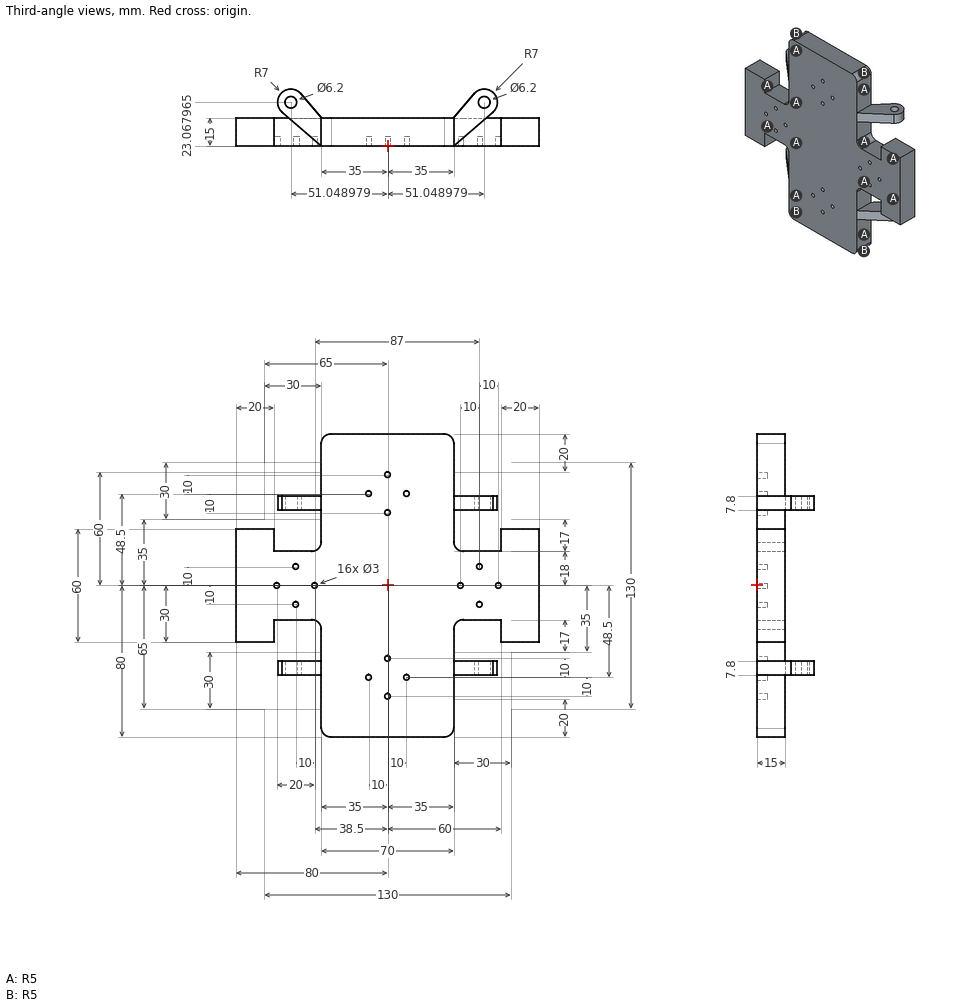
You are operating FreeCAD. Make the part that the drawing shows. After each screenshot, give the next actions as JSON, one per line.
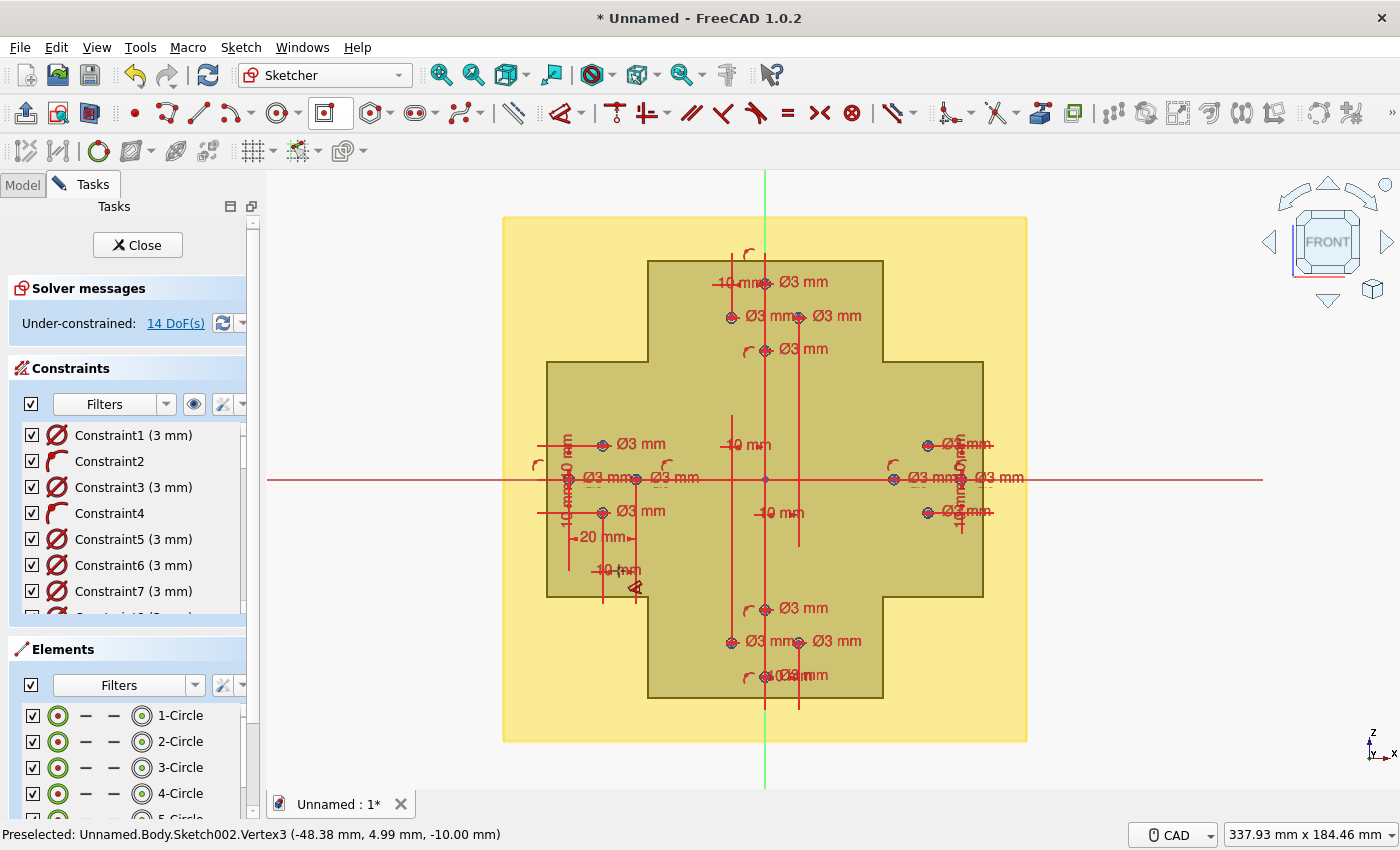
{"action": "left_click", "coordinate": [636, 480]}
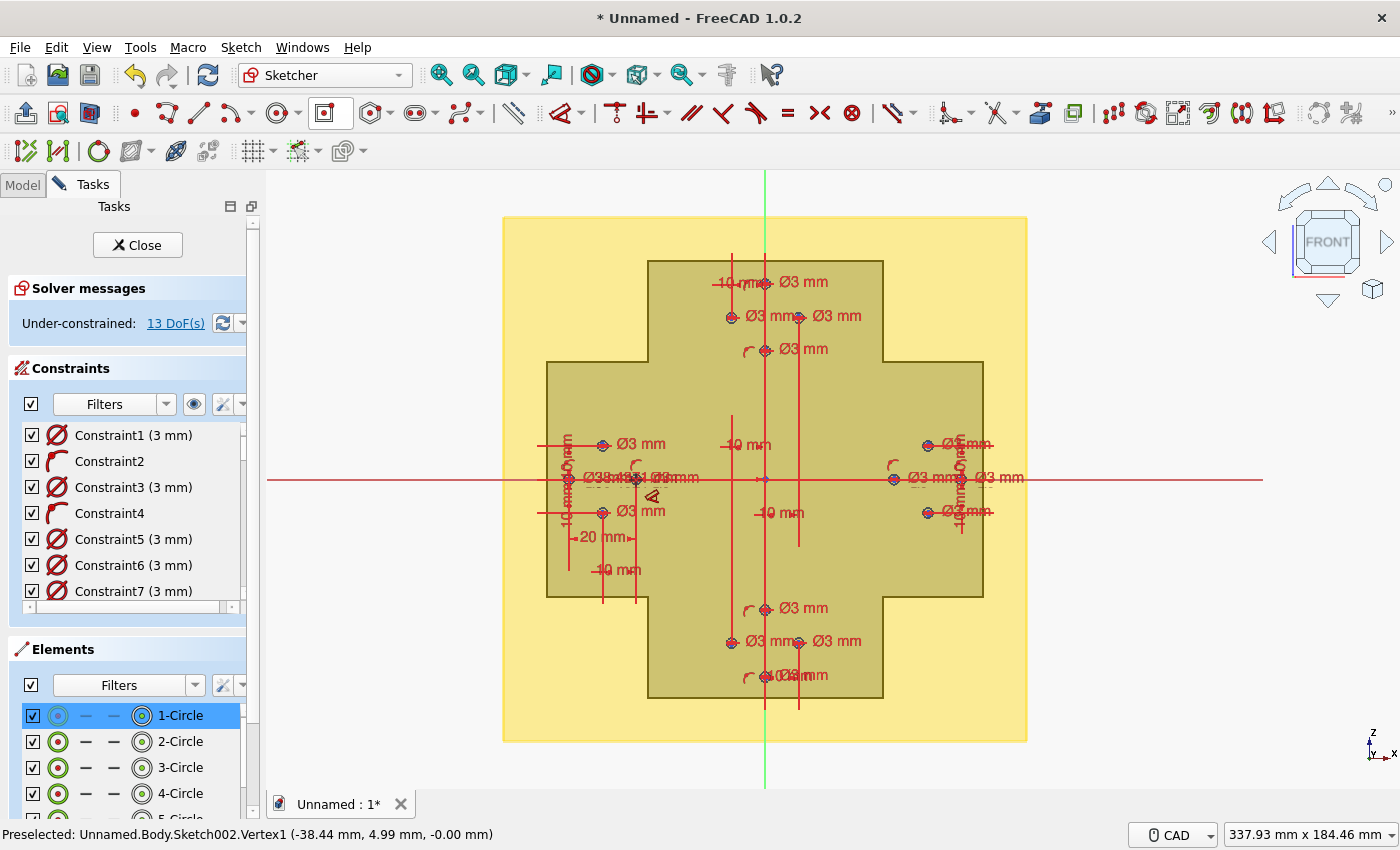
{"action": "left_click", "coordinate": [603, 446]}
{"action": "left_click", "coordinate": [619, 412]}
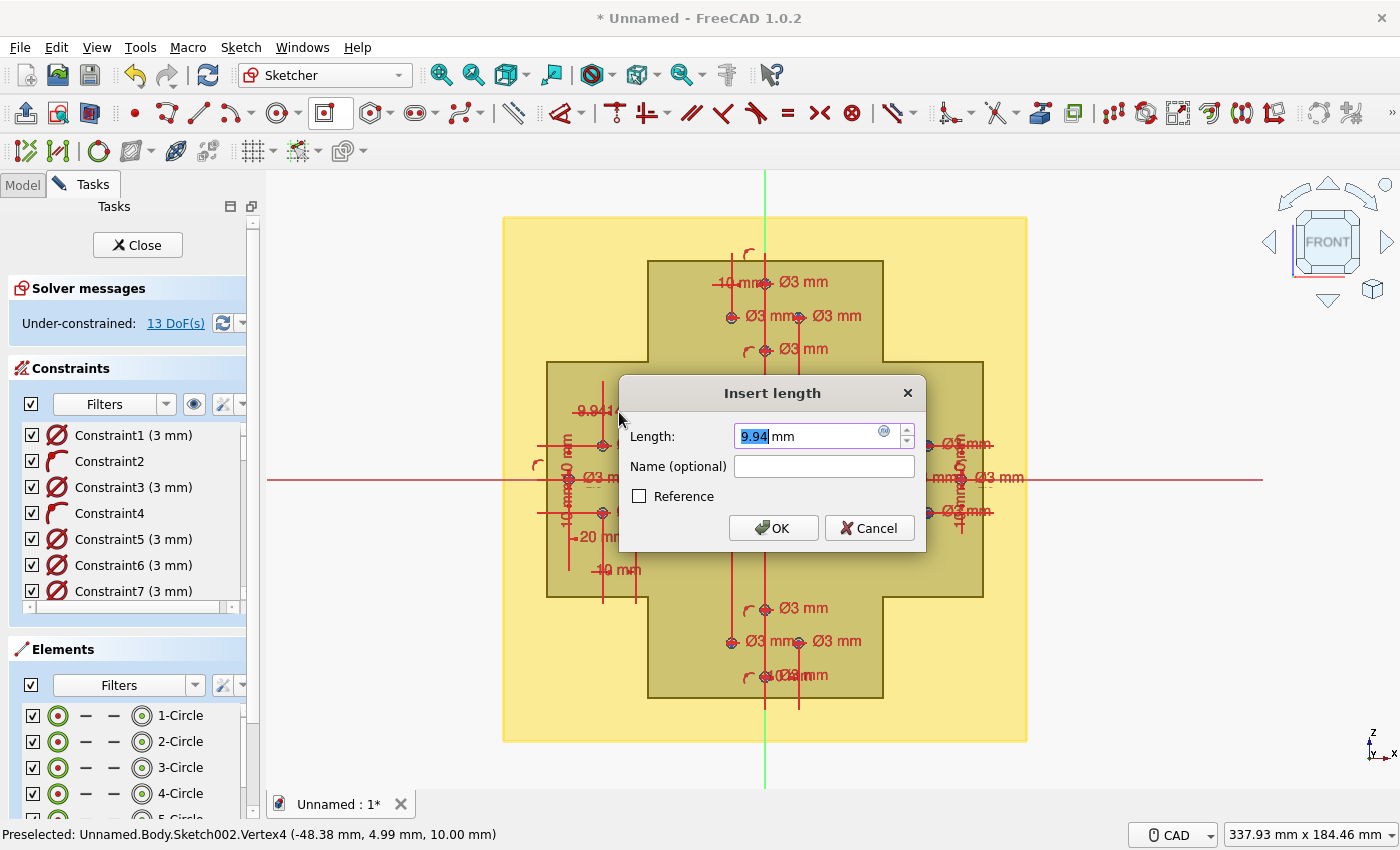
{"action": "type", "text": "10"}
{"action": "key", "text": "Return"}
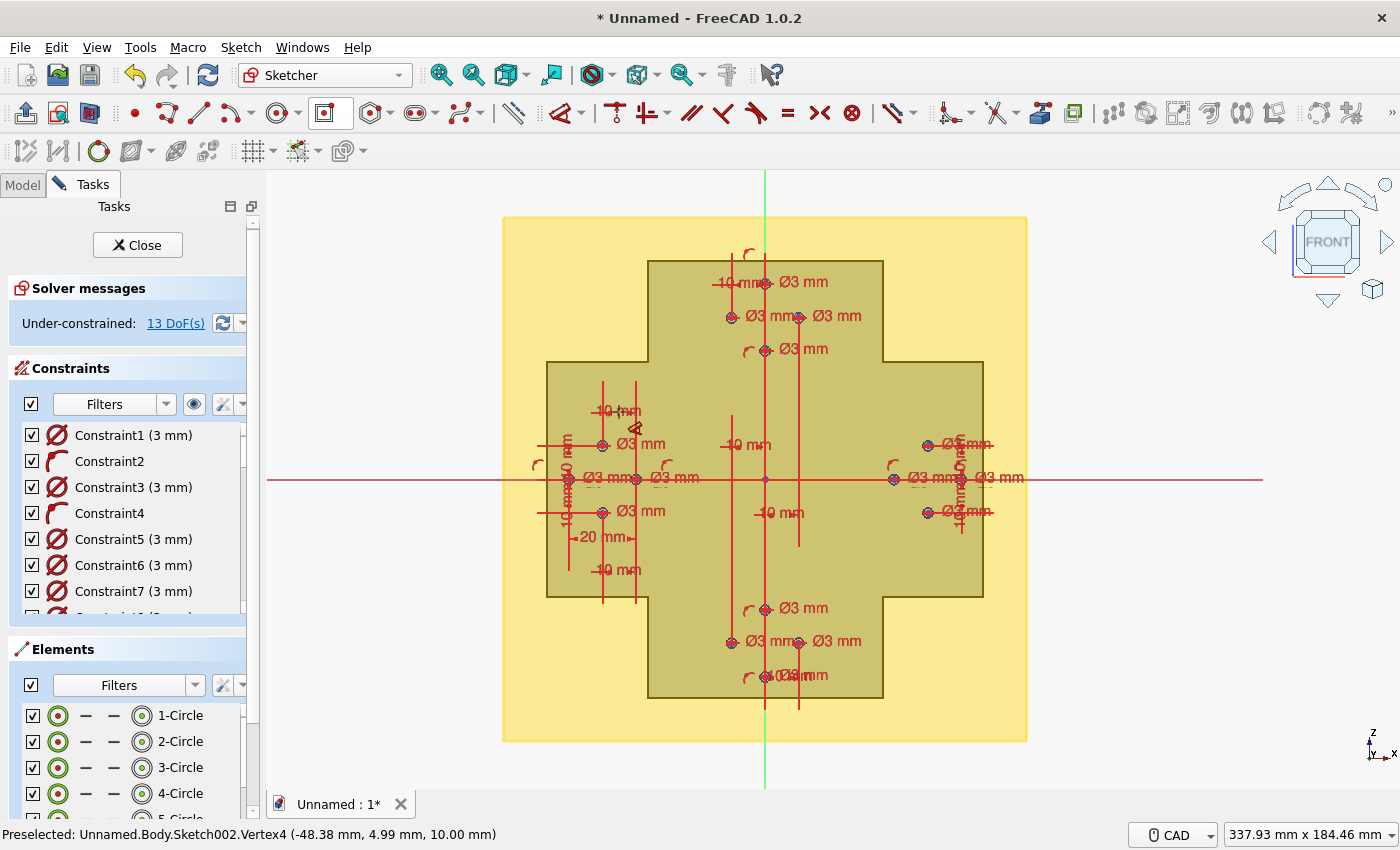
{"action": "left_click", "coordinate": [799, 643]}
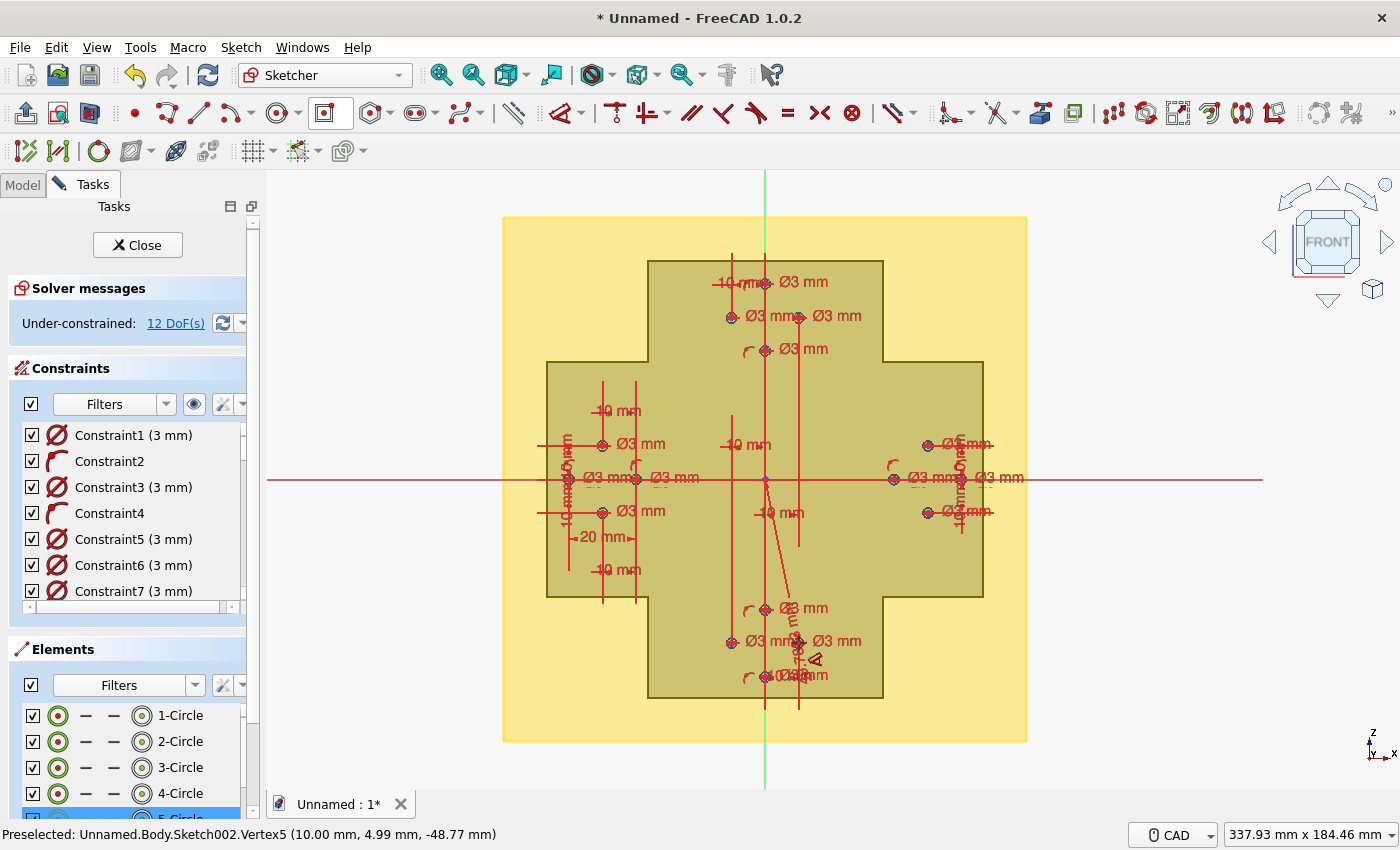
{"action": "left_click", "coordinate": [765, 610]}
{"action": "left_click", "coordinate": [833, 627]}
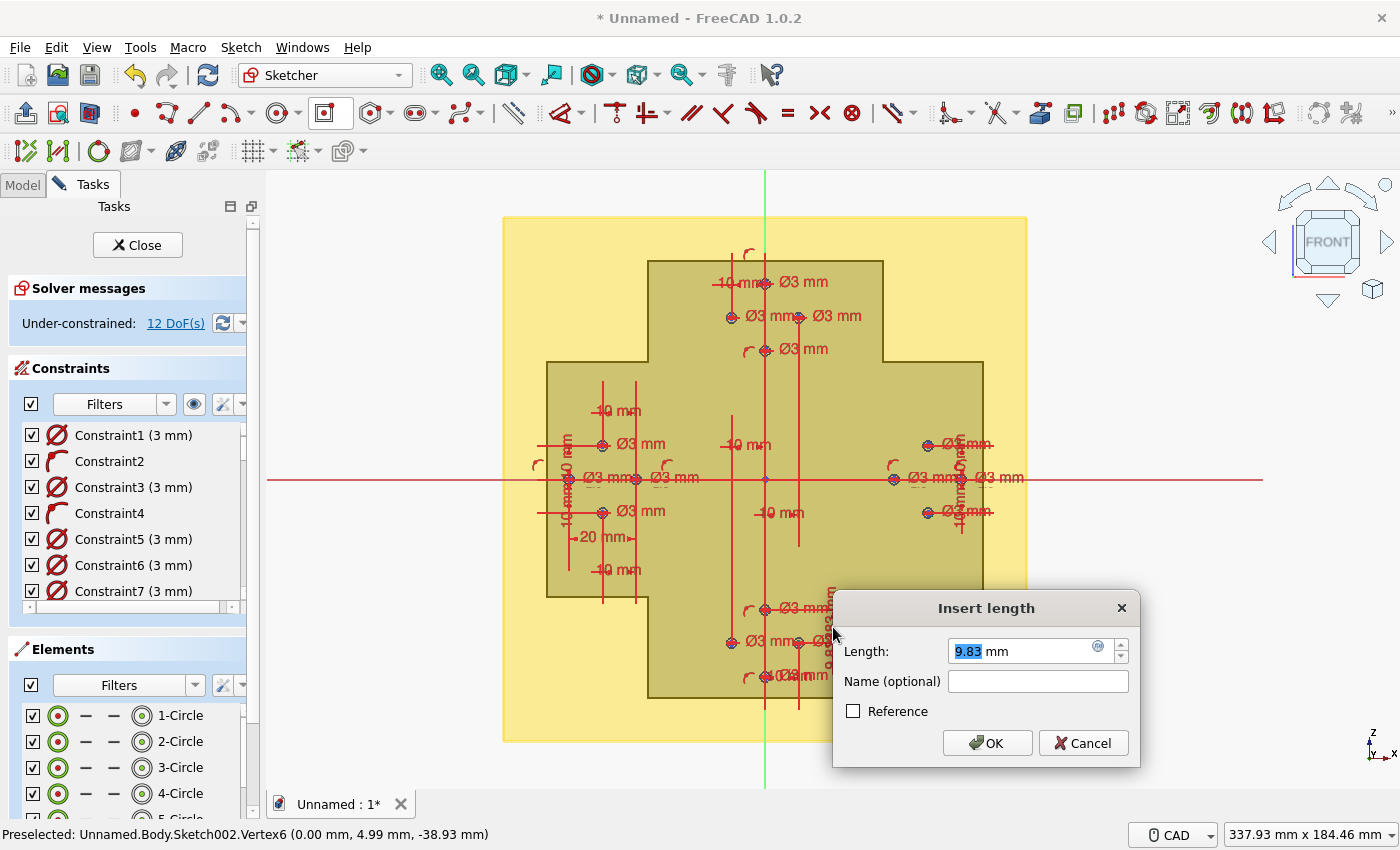
{"action": "type", "text": "10"}
{"action": "key", "text": "Return"}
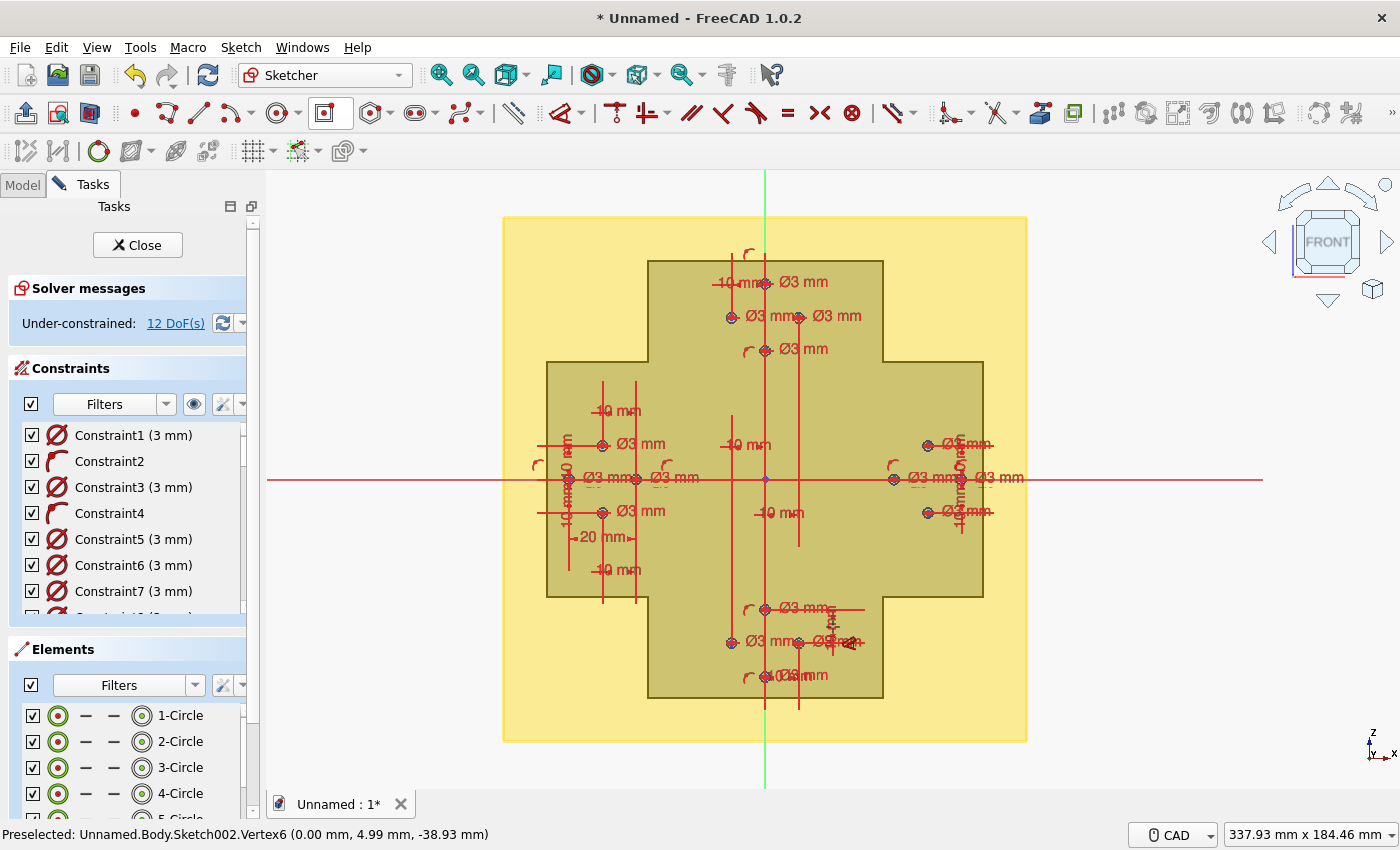
{"action": "left_click", "coordinate": [765, 610]}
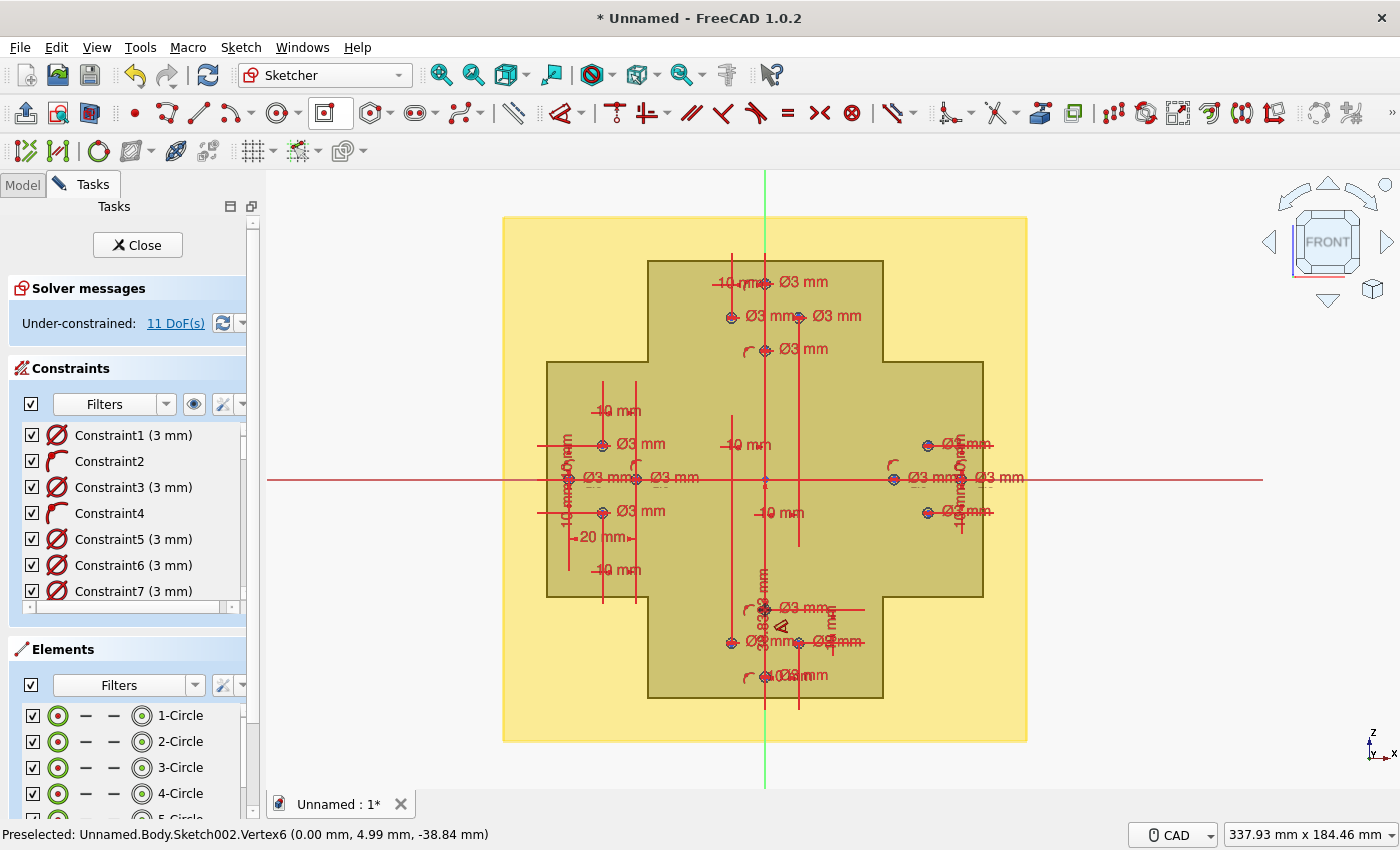
{"action": "left_click", "coordinate": [732, 643]}
{"action": "left_click", "coordinate": [698, 627]}